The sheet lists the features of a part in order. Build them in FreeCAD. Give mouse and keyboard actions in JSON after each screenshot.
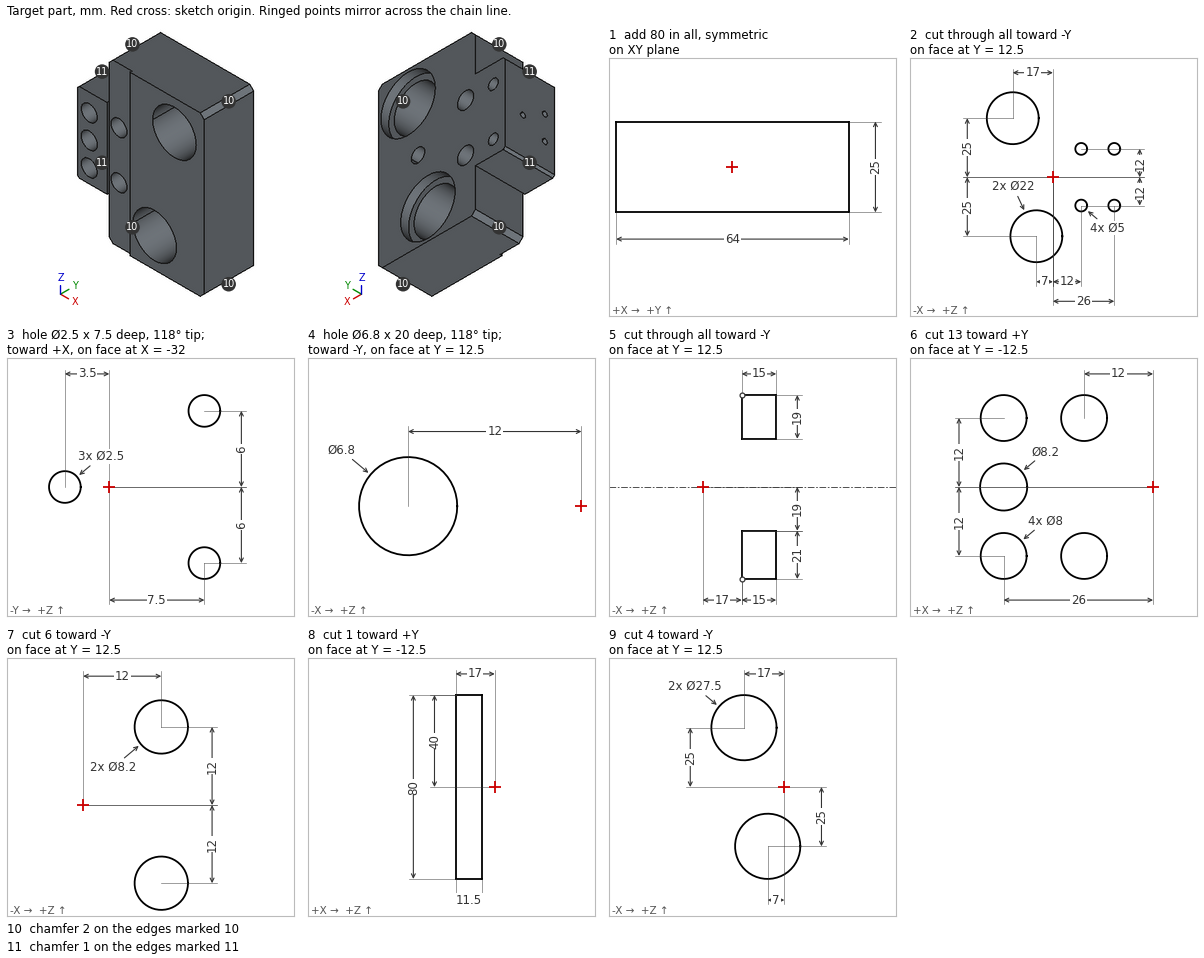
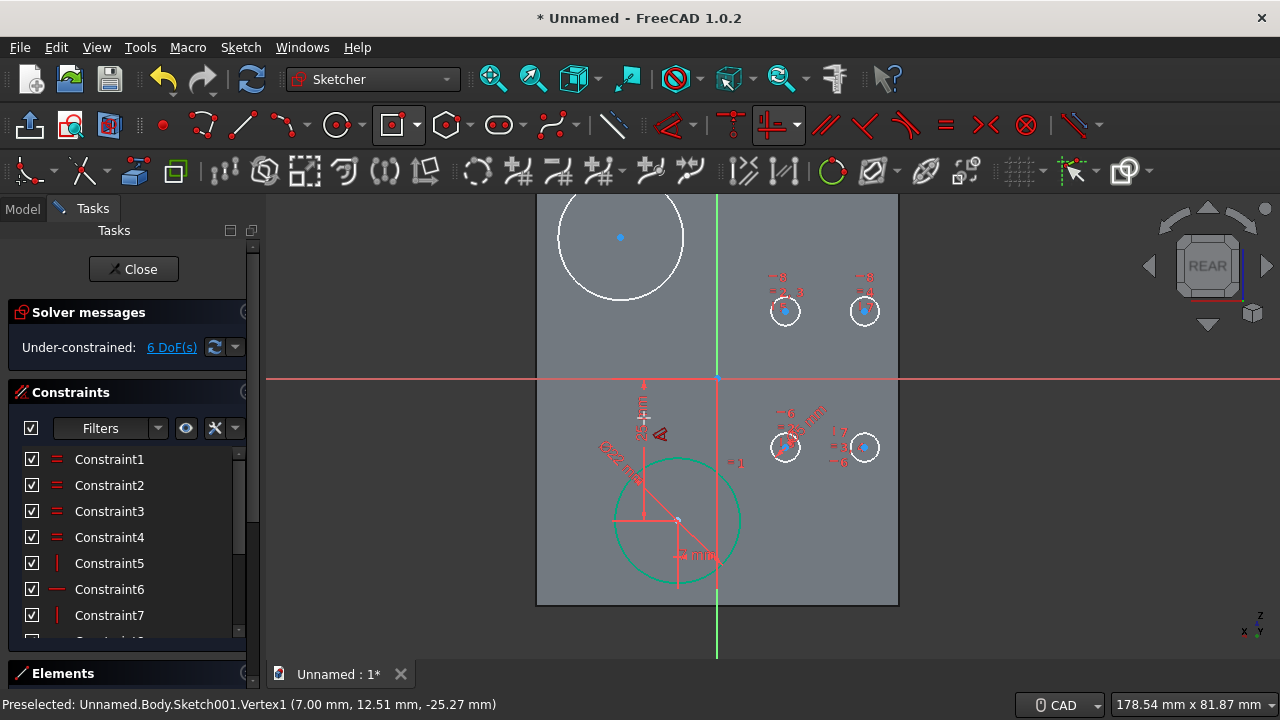
{"action": "left_click", "coordinate": [621, 238]}
{"action": "left_click", "coordinate": [691, 485]}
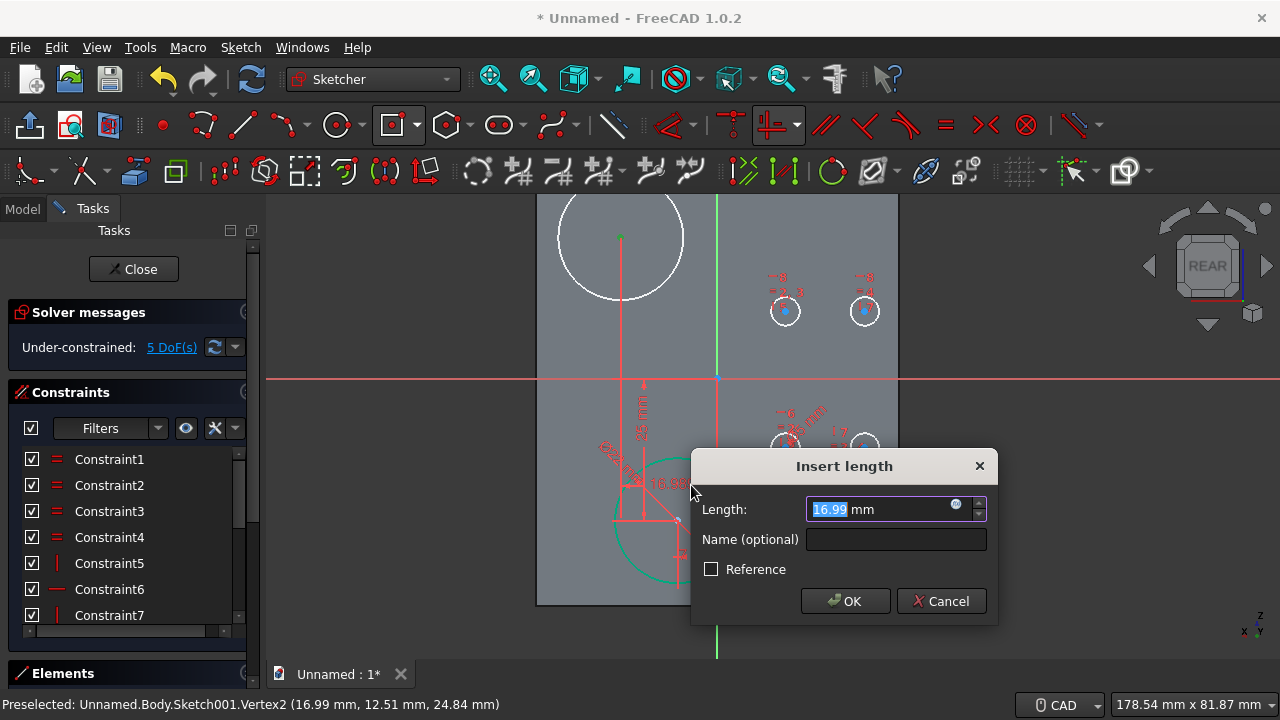
{"action": "type", "text": "17"}
{"action": "key", "text": "Return"}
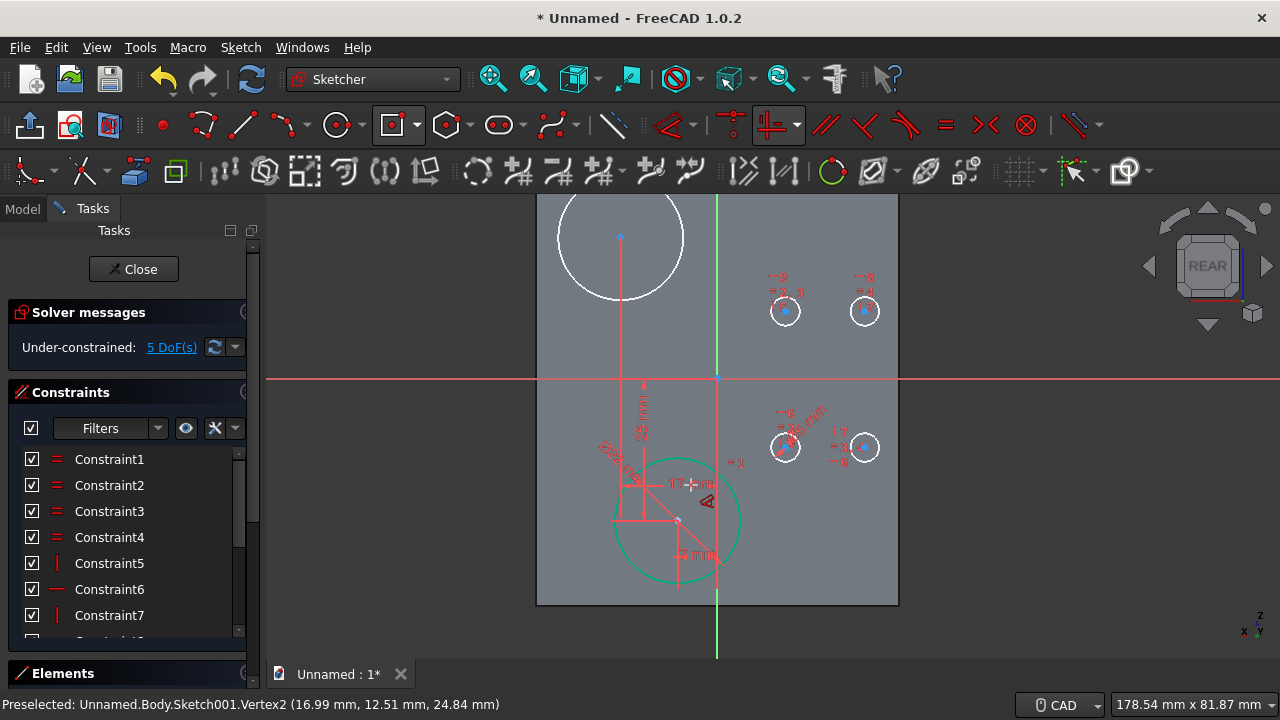
{"action": "left_click", "coordinate": [621, 238]}
{"action": "left_click", "coordinate": [587, 308]}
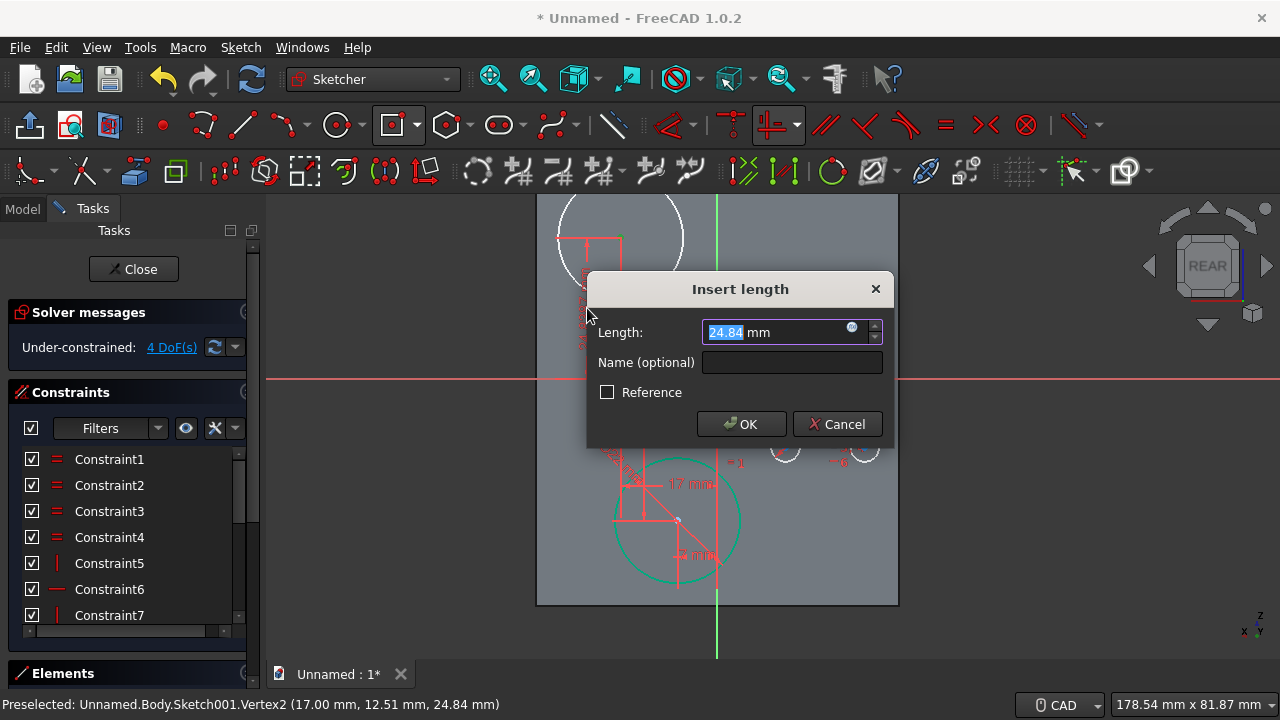
{"action": "type", "text": "25"}
{"action": "key", "text": "Return"}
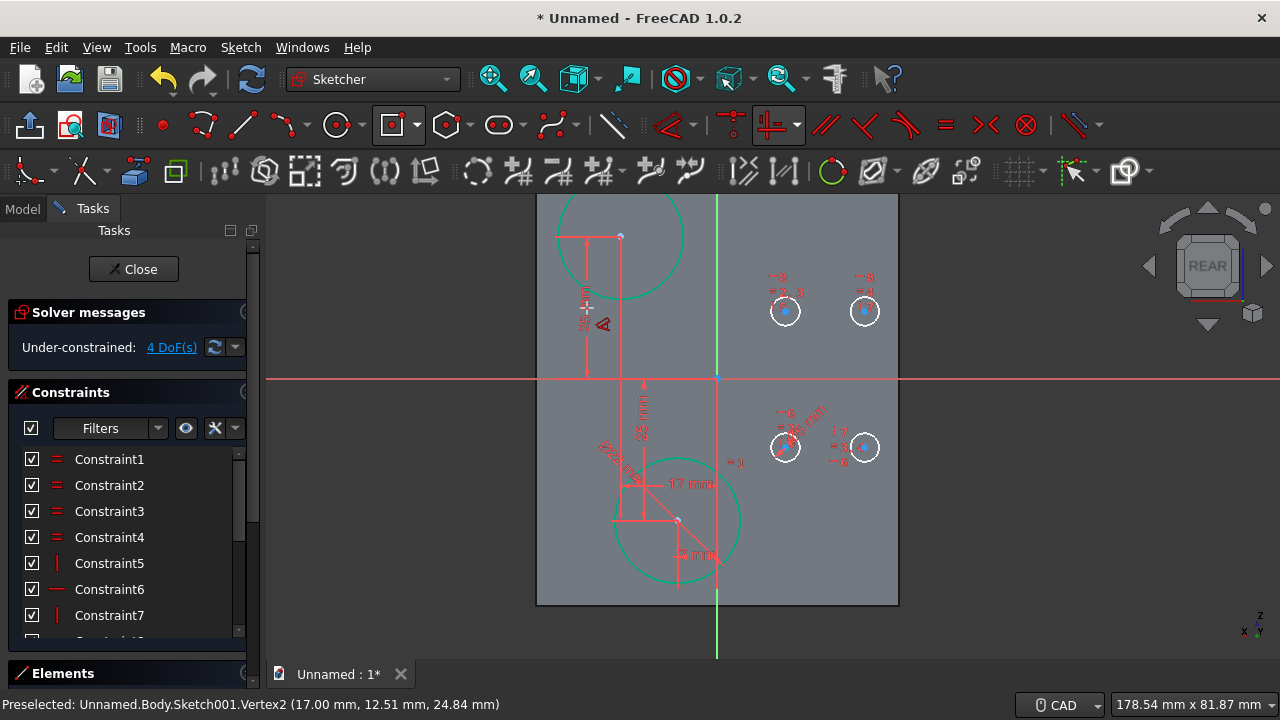
{"action": "left_click", "coordinate": [785, 448]}
{"action": "left_click", "coordinate": [767, 482]}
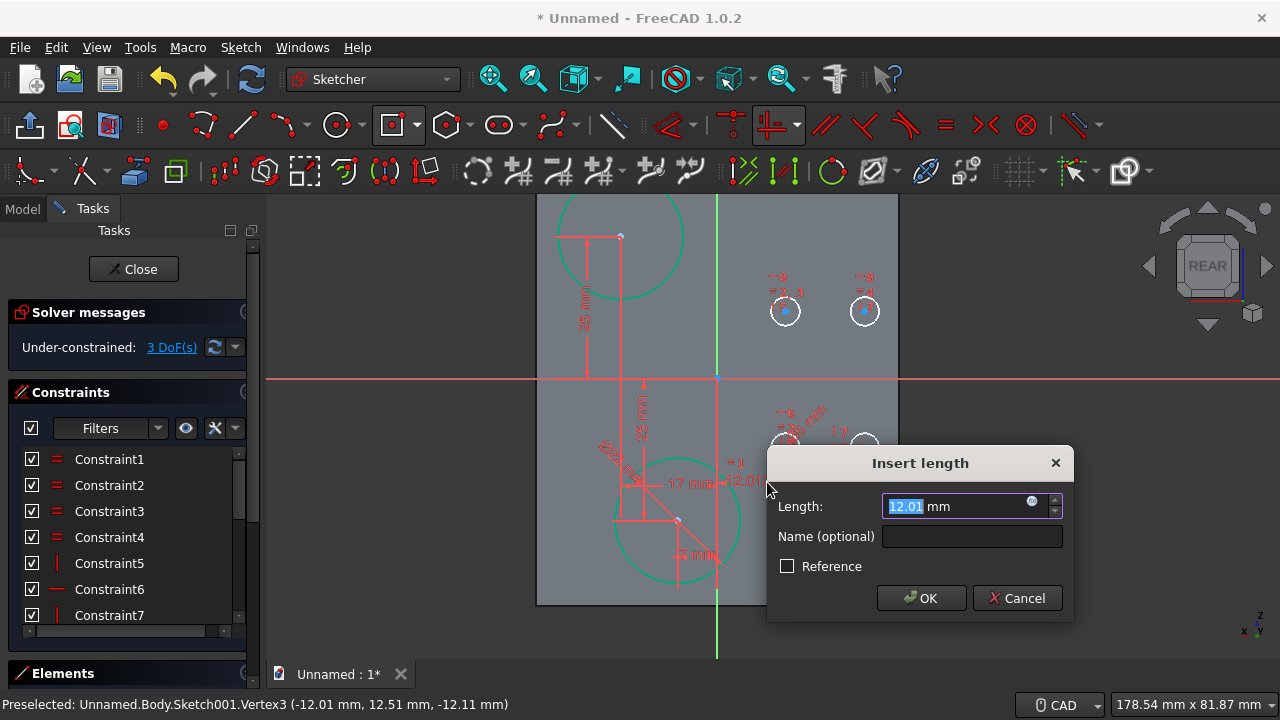
{"action": "type", "text": "12"}
{"action": "key", "text": "Return"}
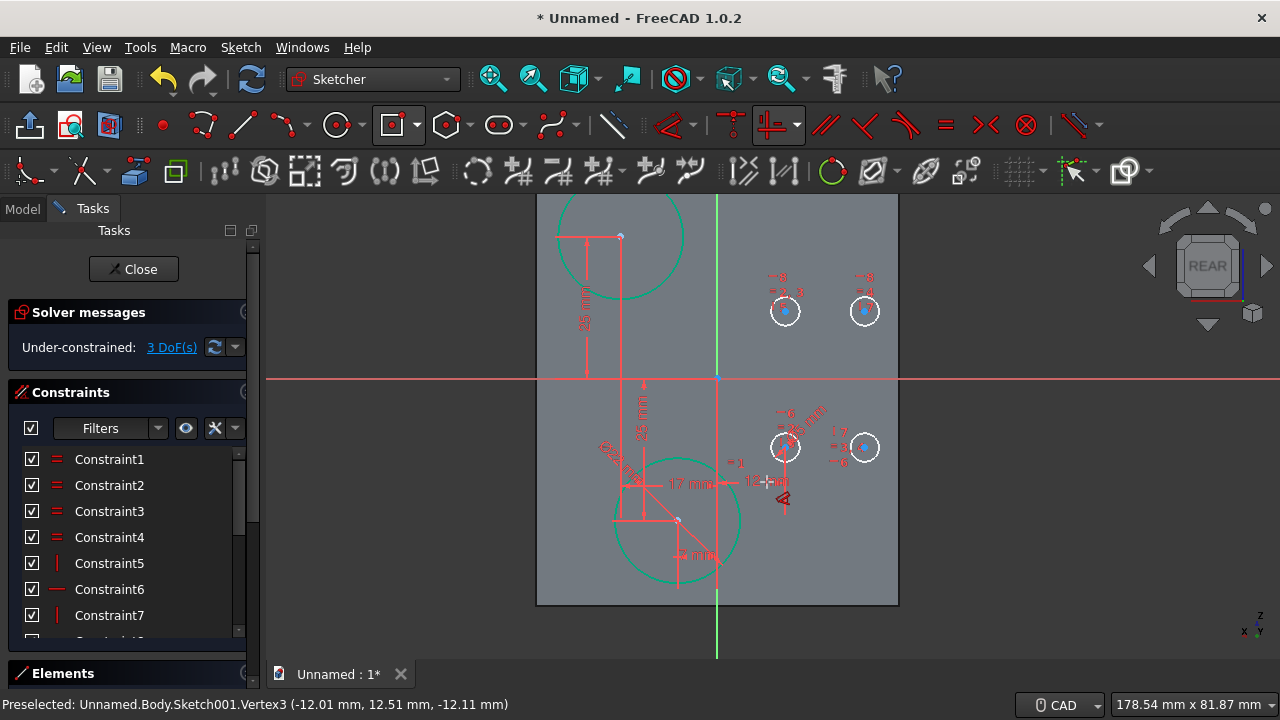
{"action": "left_click", "coordinate": [785, 448]}
{"action": "left_click", "coordinate": [819, 397]}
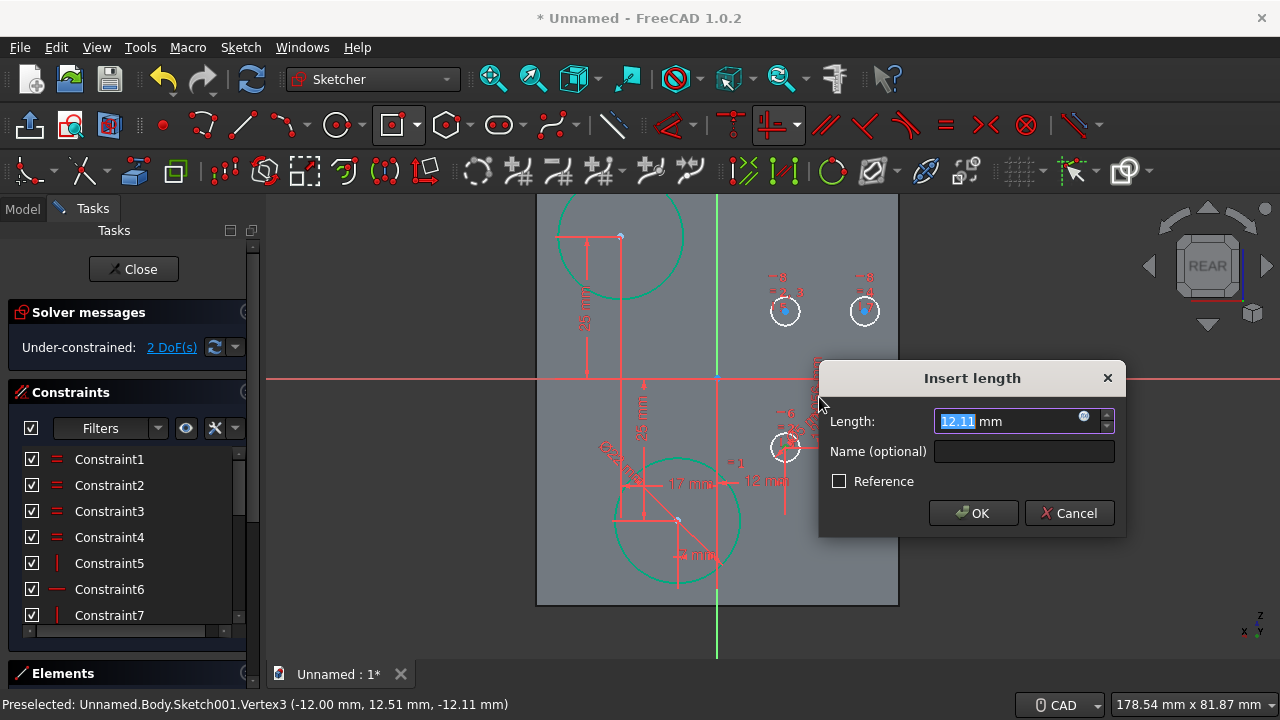
{"action": "type", "text": "12"}
{"action": "key", "text": "Return"}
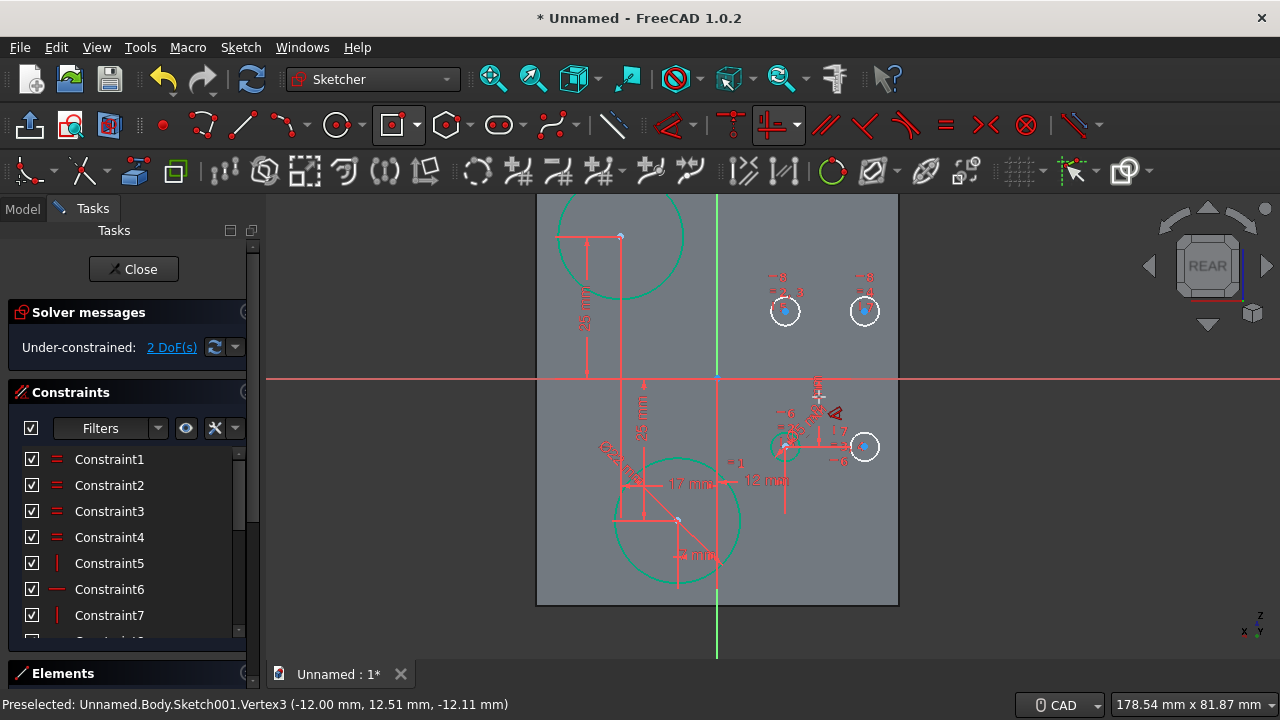
{"action": "left_click", "coordinate": [785, 311]}
{"action": "left_click", "coordinate": [819, 345]}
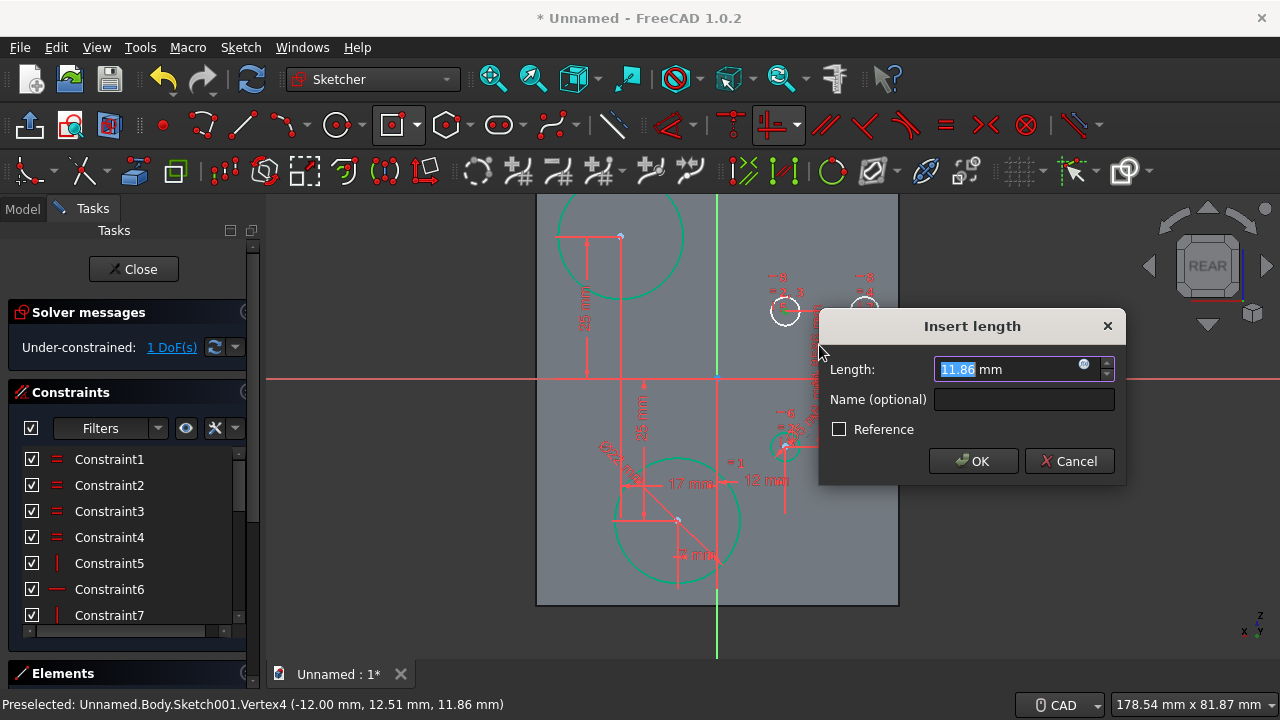
{"action": "type", "text": "12"}
{"action": "key", "text": "Return"}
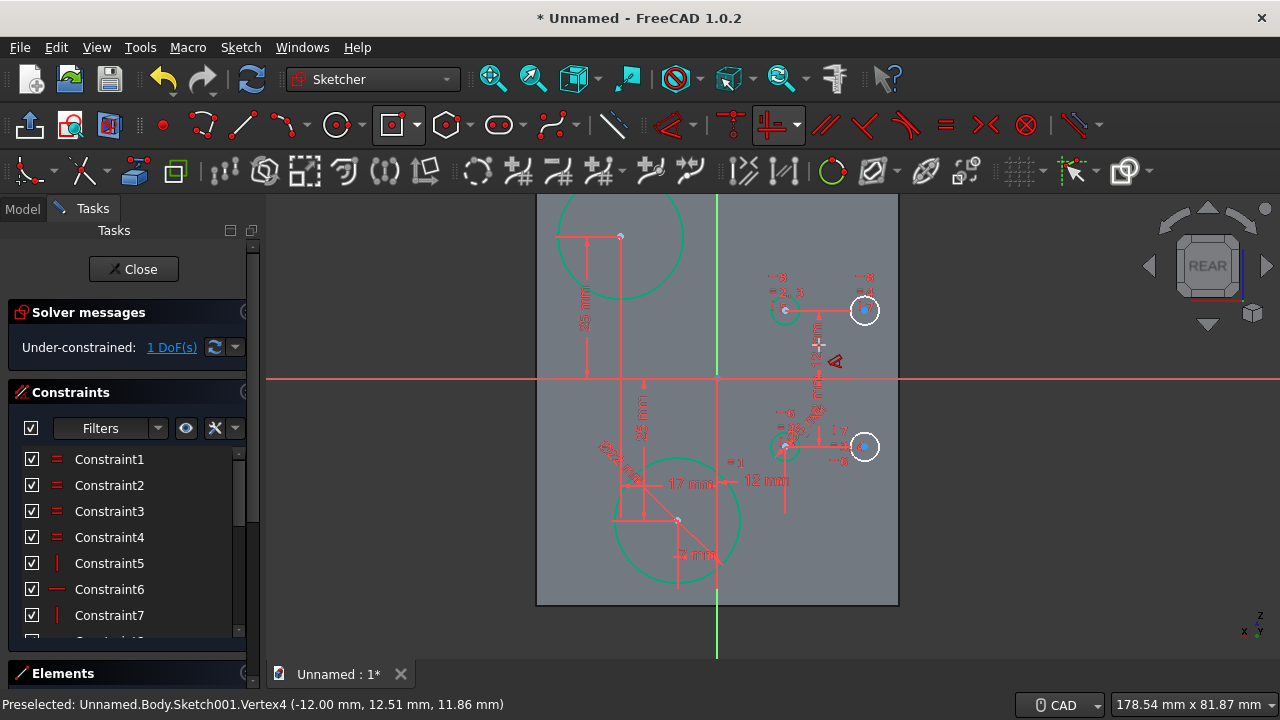
{"action": "left_click", "coordinate": [865, 447]}
{"action": "left_click", "coordinate": [843, 481]}